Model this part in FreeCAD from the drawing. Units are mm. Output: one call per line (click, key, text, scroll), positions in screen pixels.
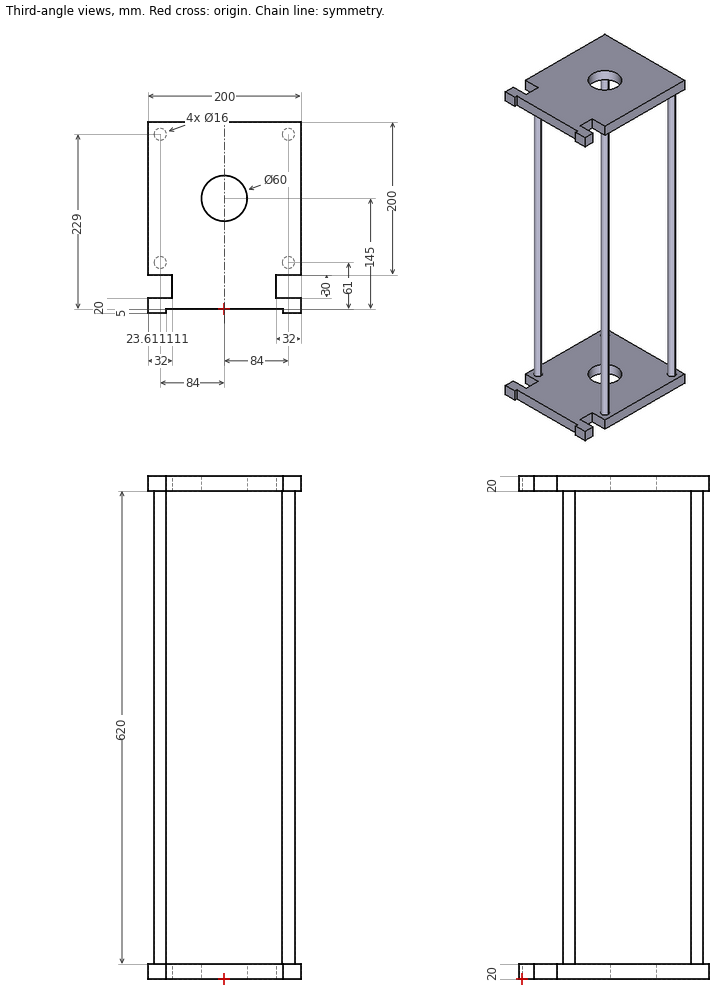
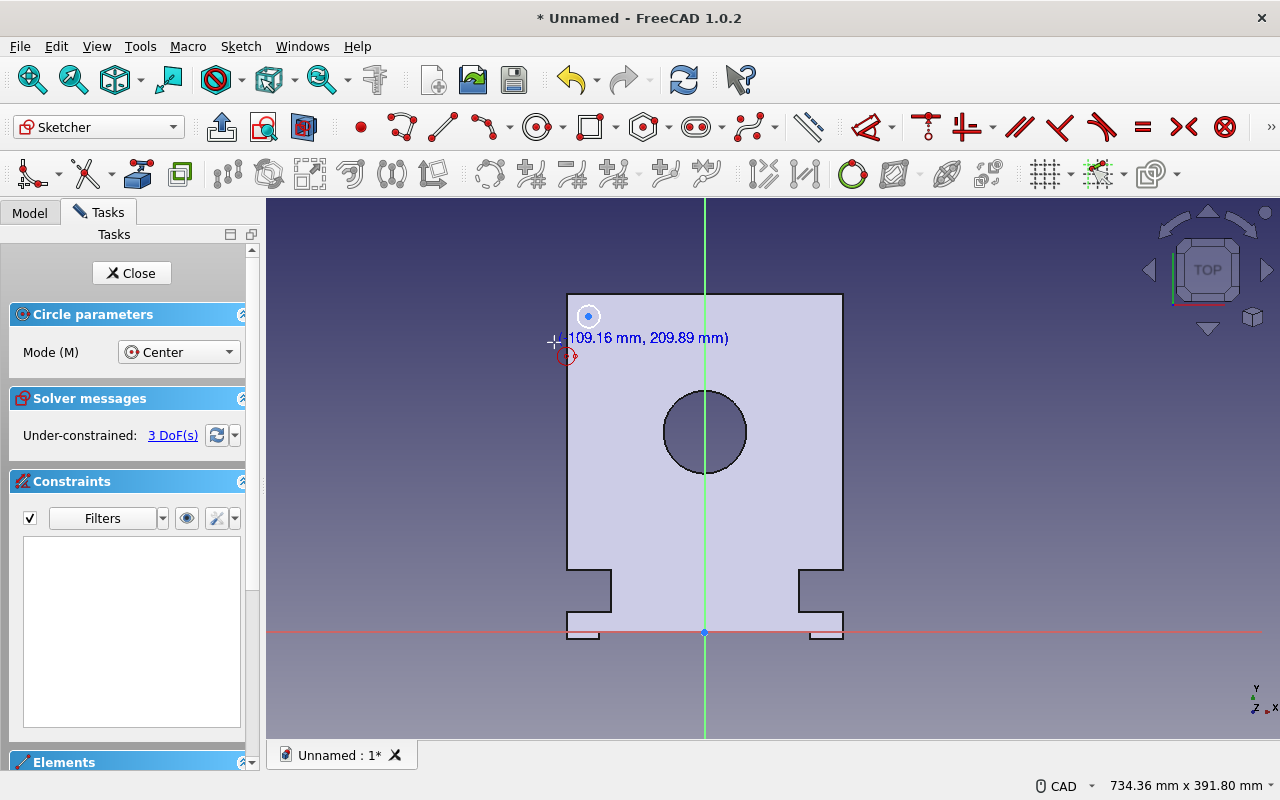
scroll(821, 316, up, 4)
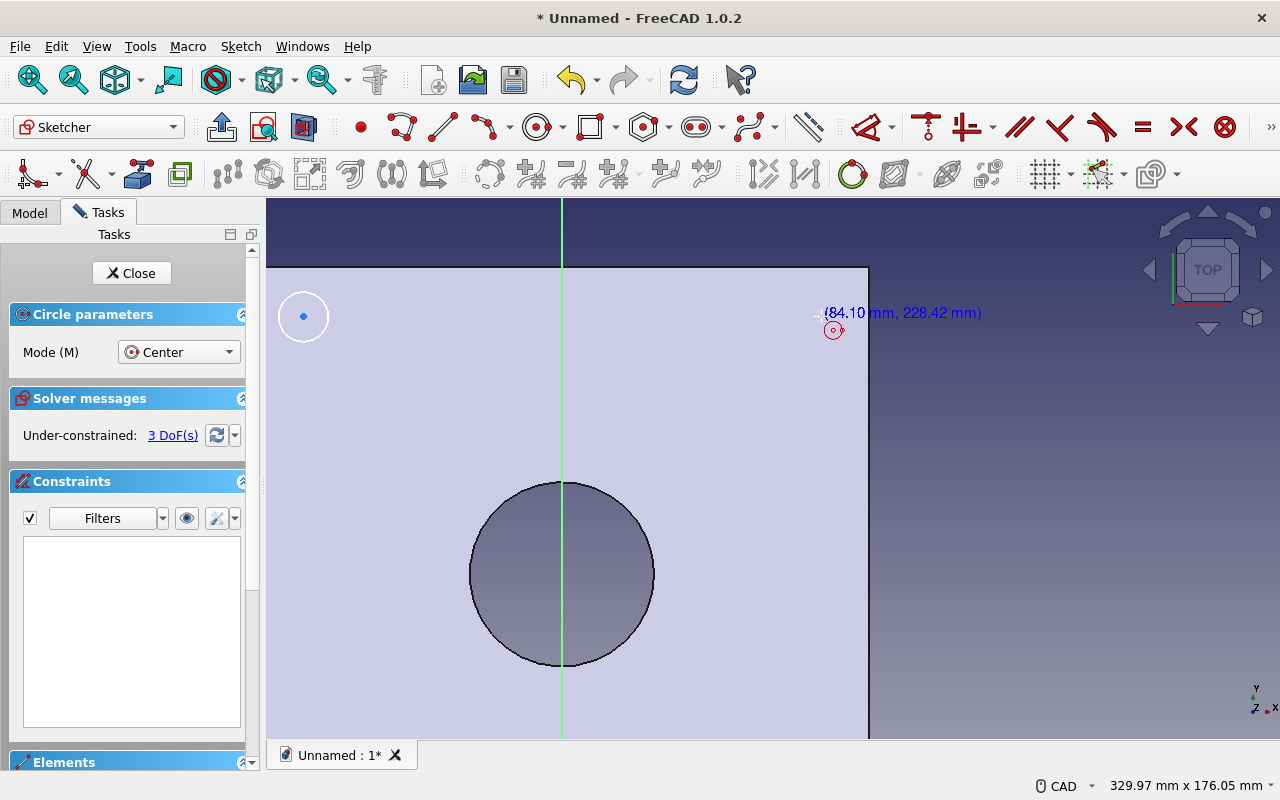
click(820, 316)
click(837, 299)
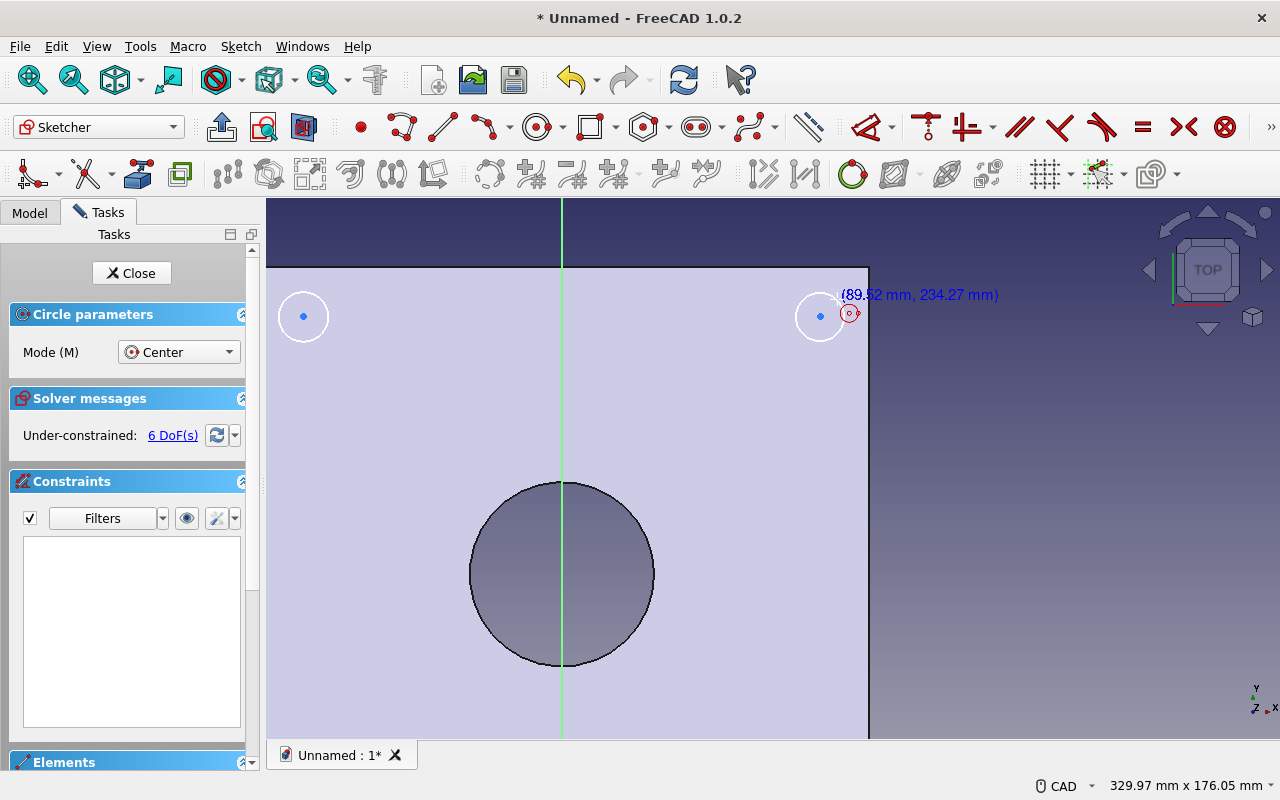
scroll(821, 316, down, 4)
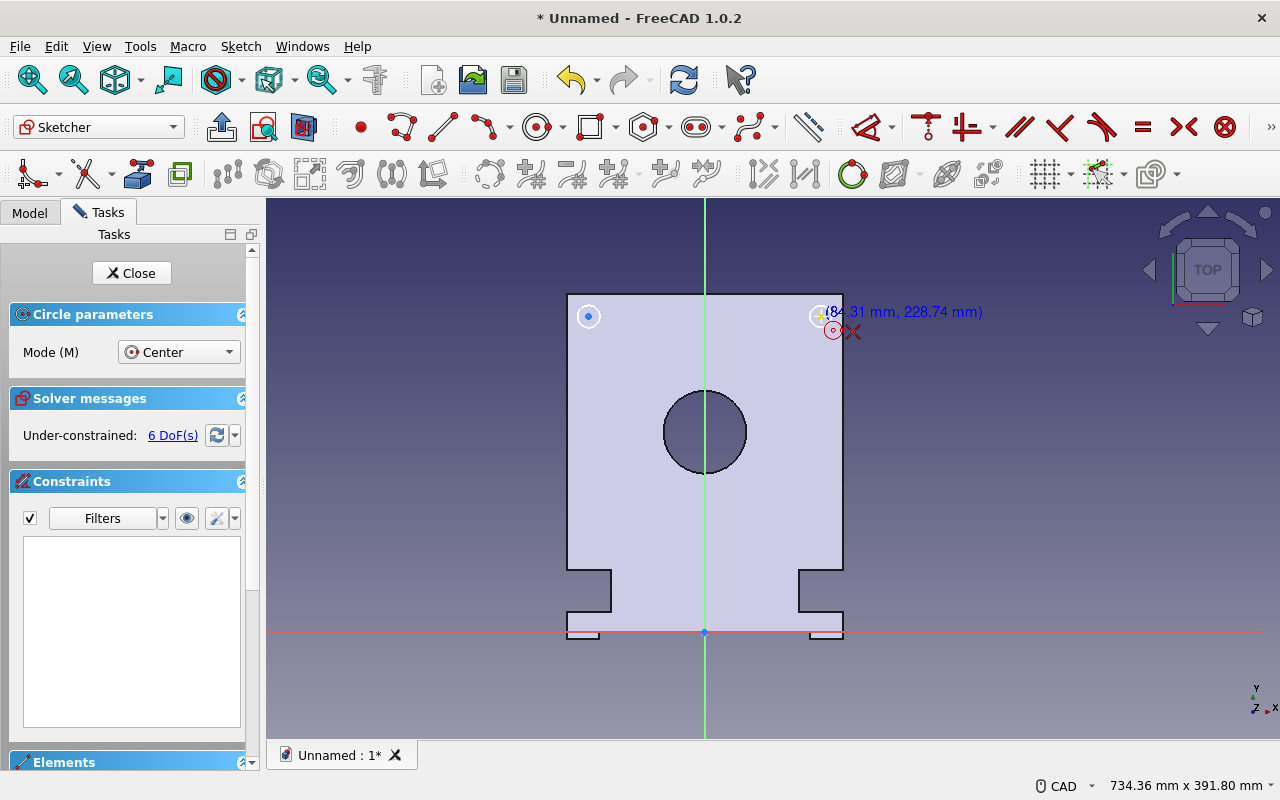
scroll(821, 548, up, 4)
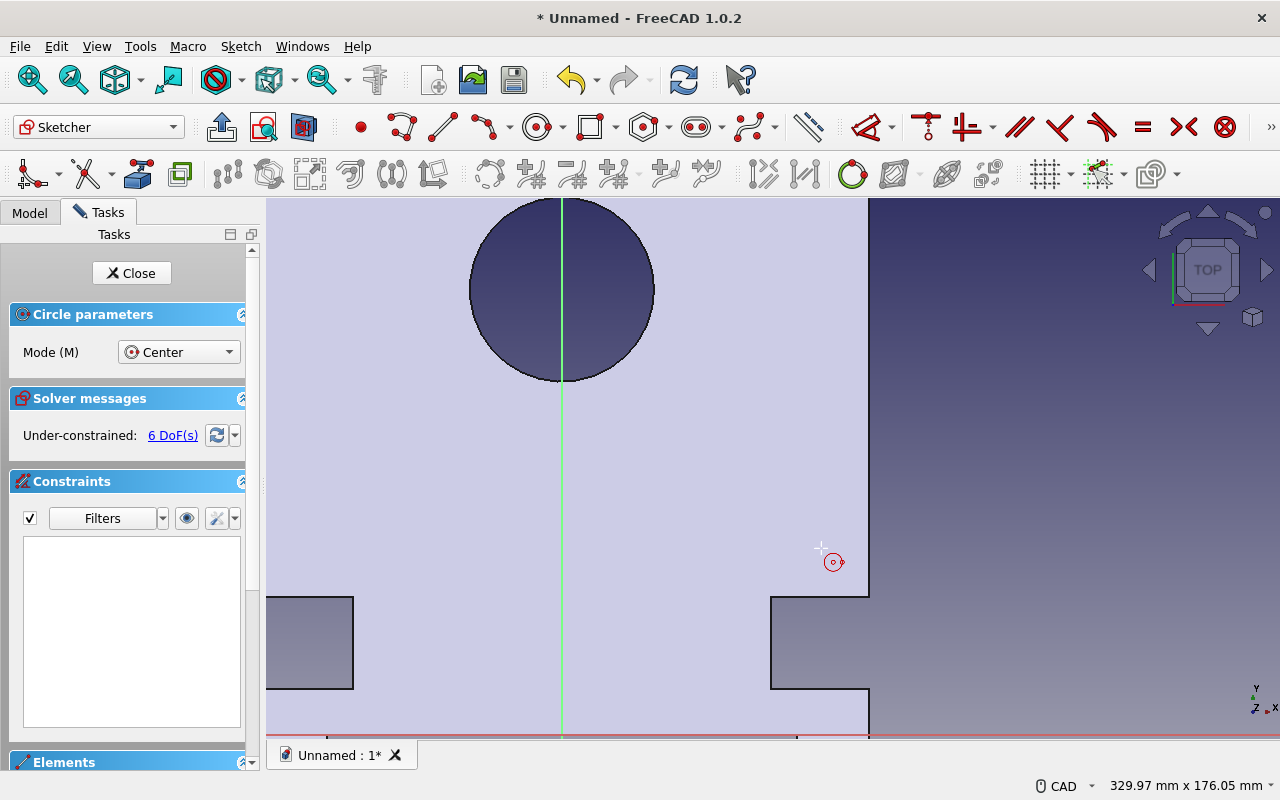
click(820, 548)
click(837, 530)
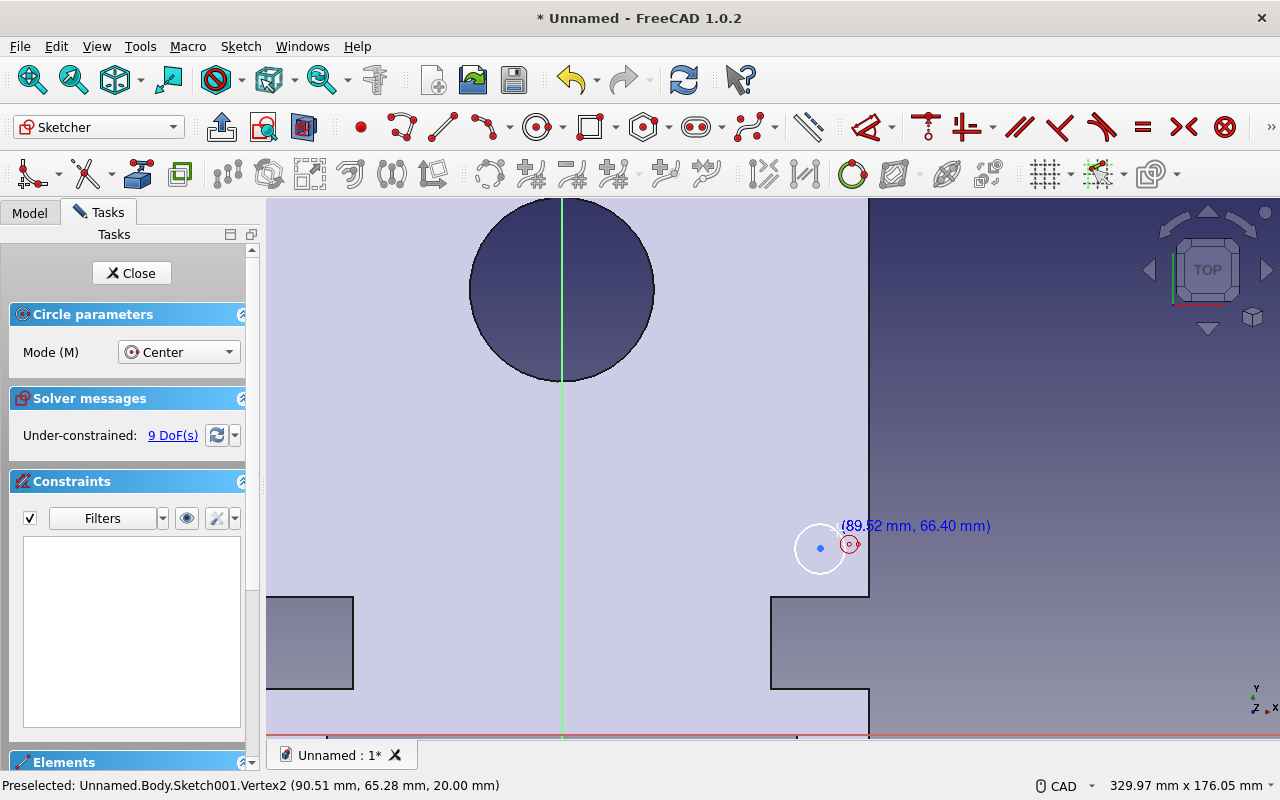
click(304, 548)
click(321, 530)
key(Escape)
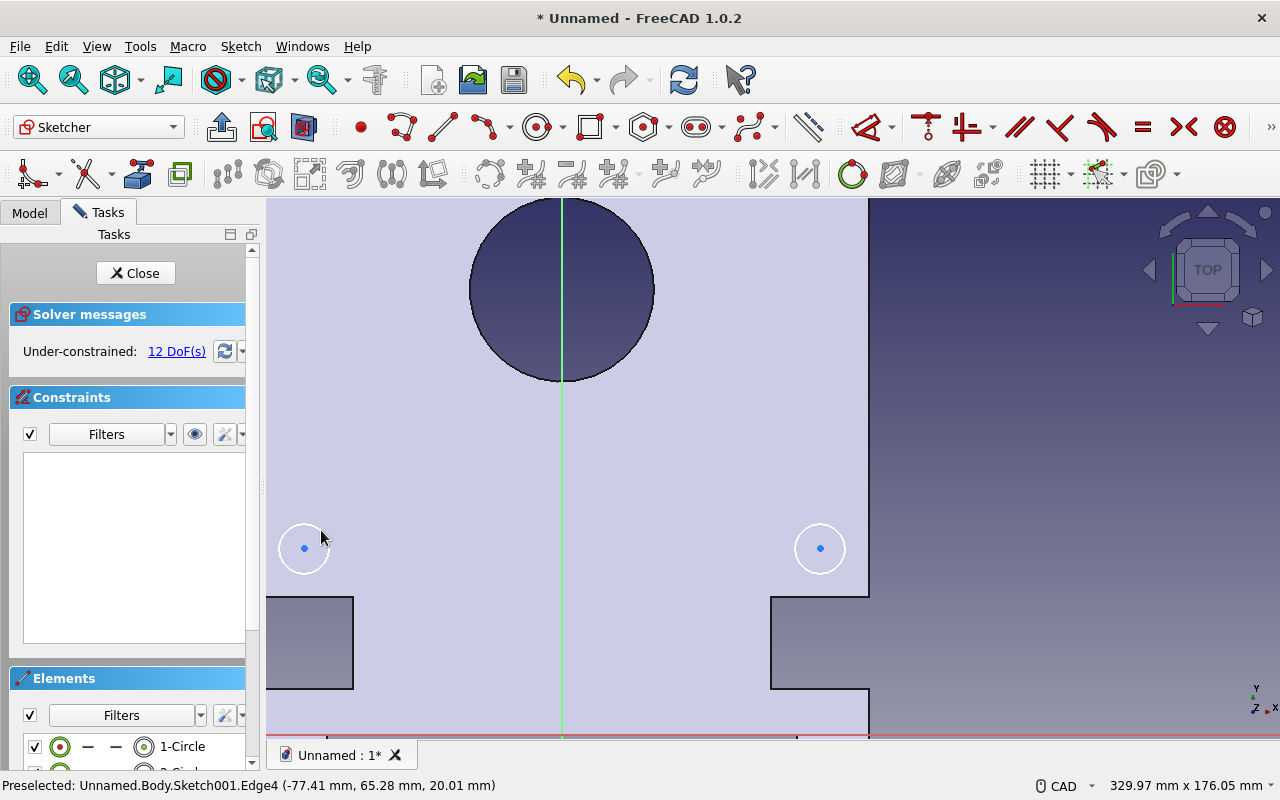
scroll(821, 548, down, 4)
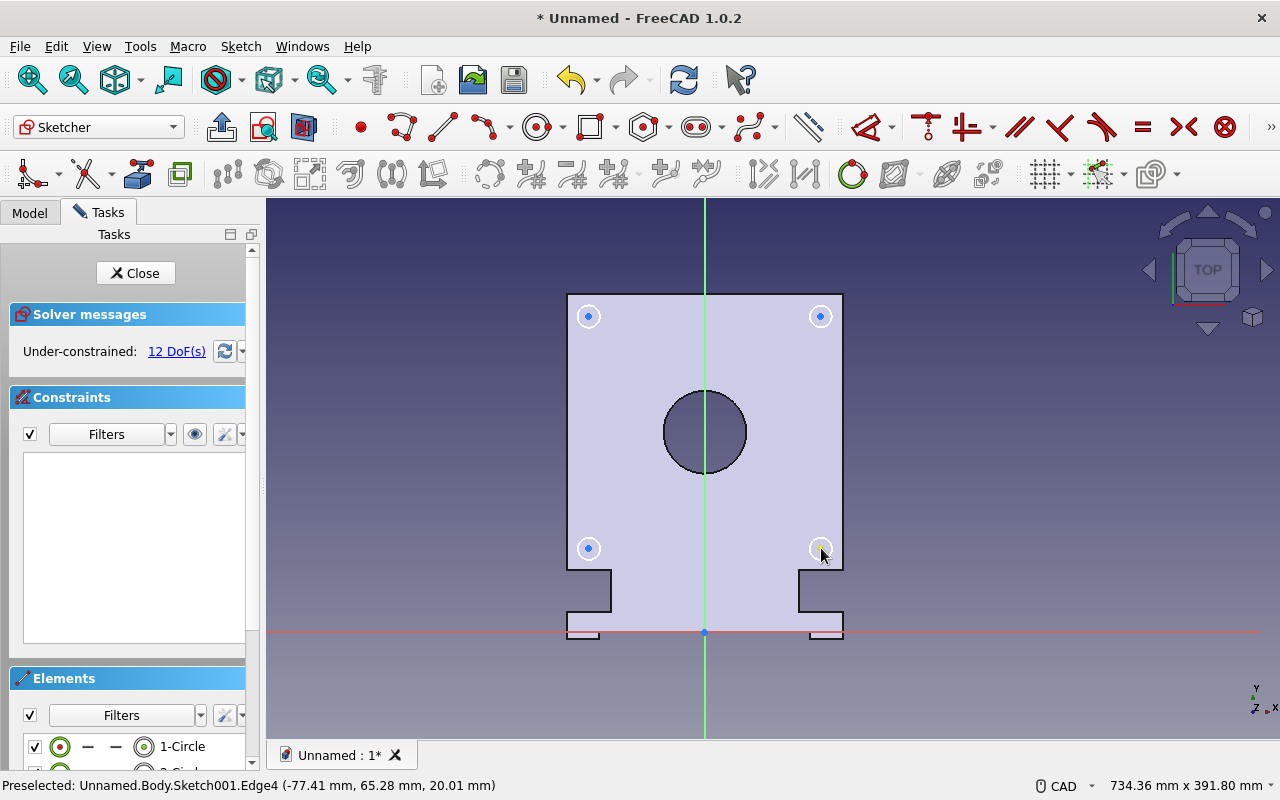
scroll(597, 309, up, 2)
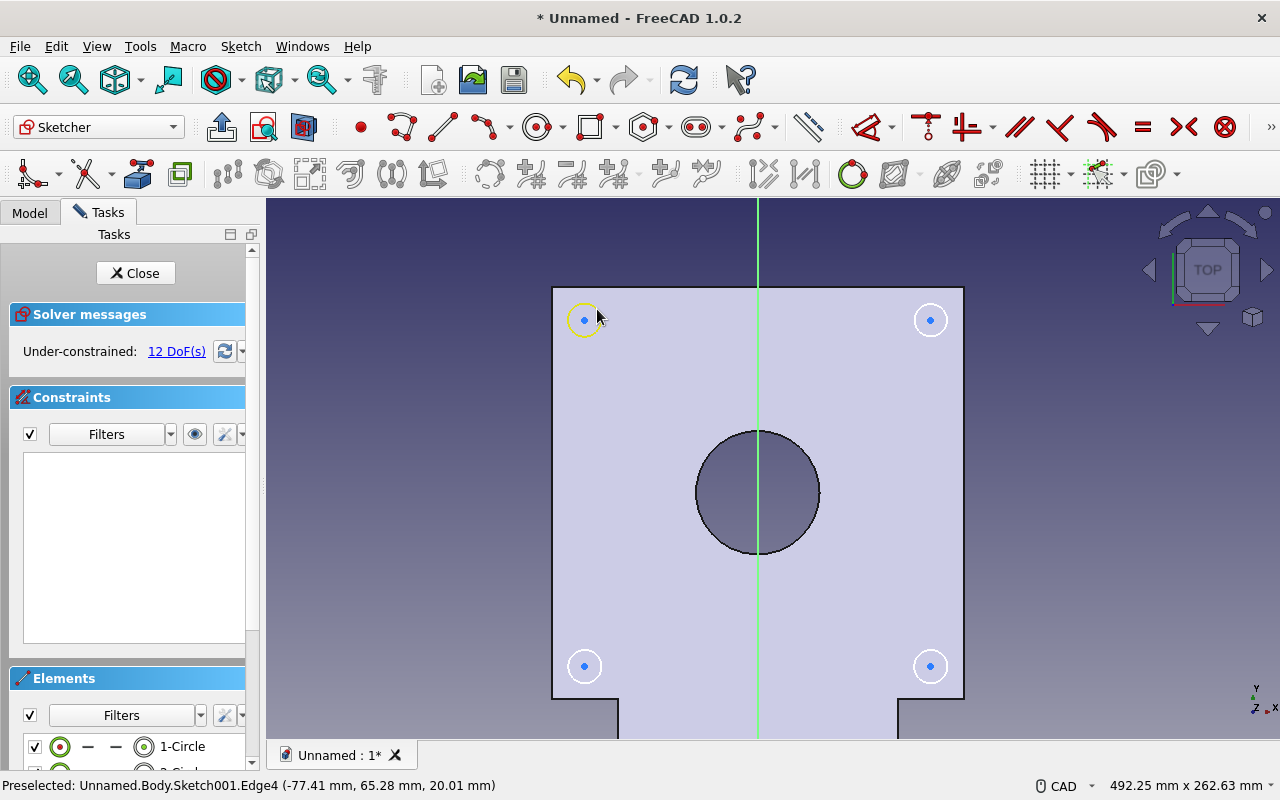
click(596, 308)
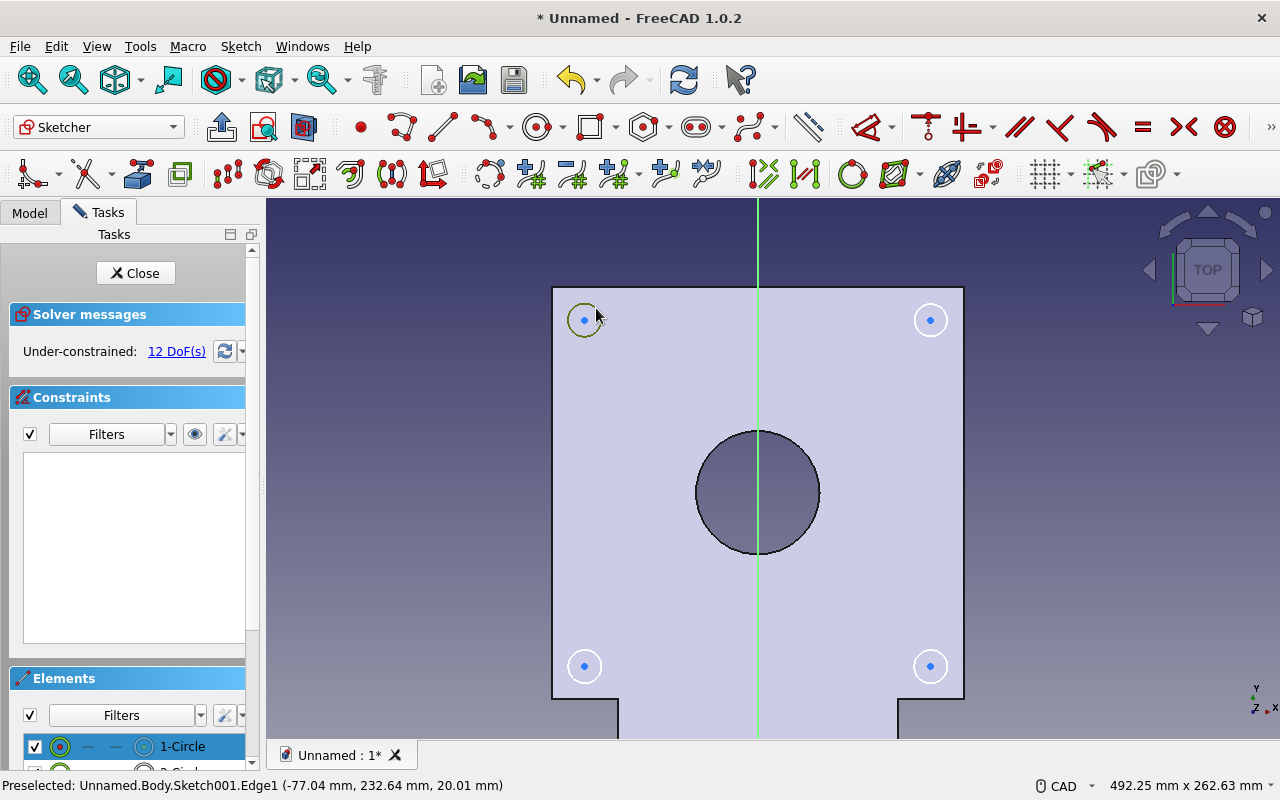
click(942, 309)